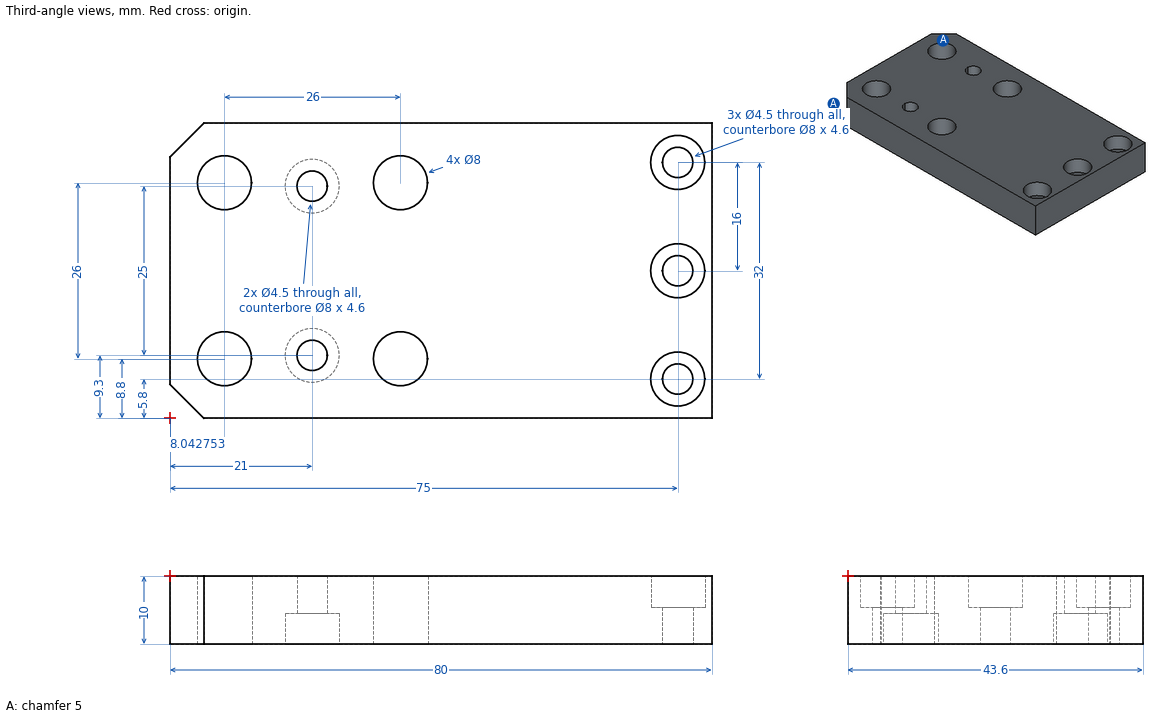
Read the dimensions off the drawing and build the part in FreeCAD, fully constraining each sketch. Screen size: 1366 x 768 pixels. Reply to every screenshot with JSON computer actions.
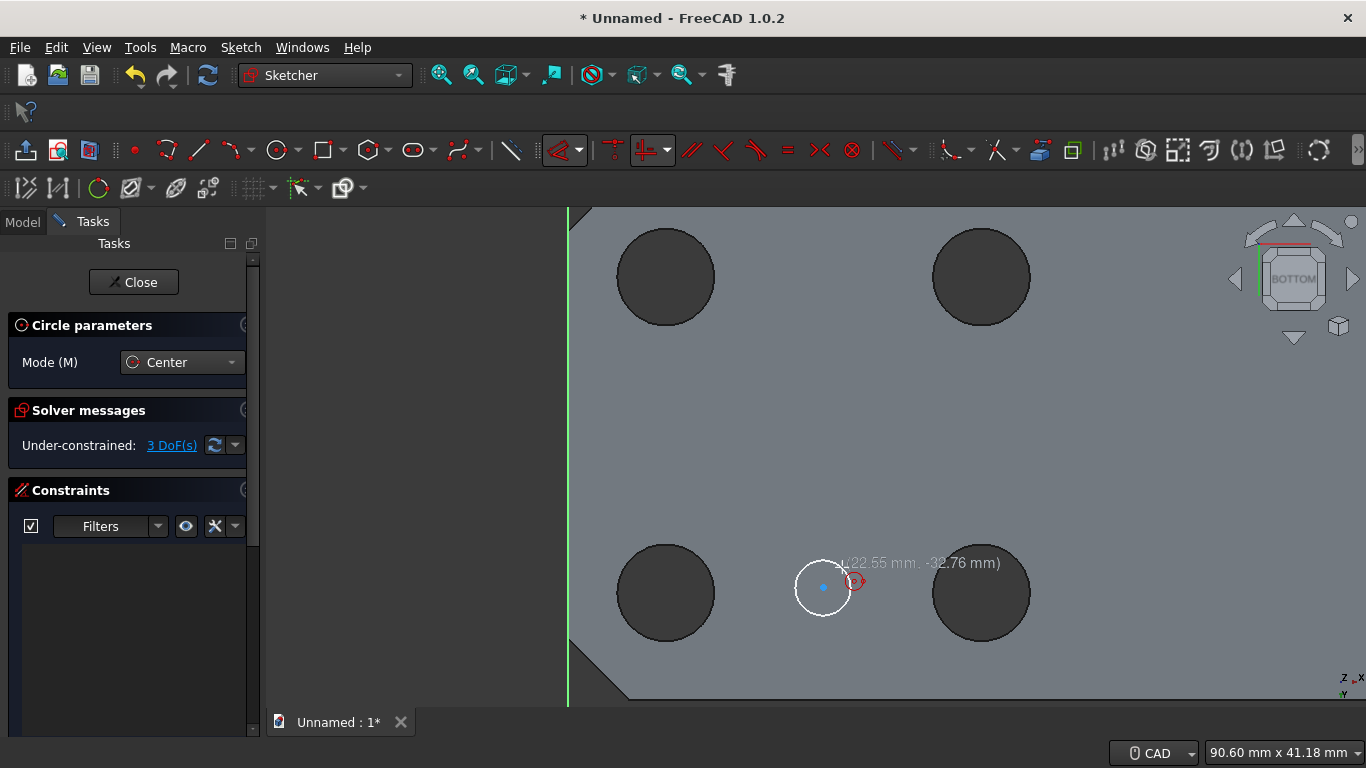
{"action": "left_click", "coordinate": [823, 283]}
{"action": "left_click", "coordinate": [842, 264]}
{"action": "key", "text": "Escape"}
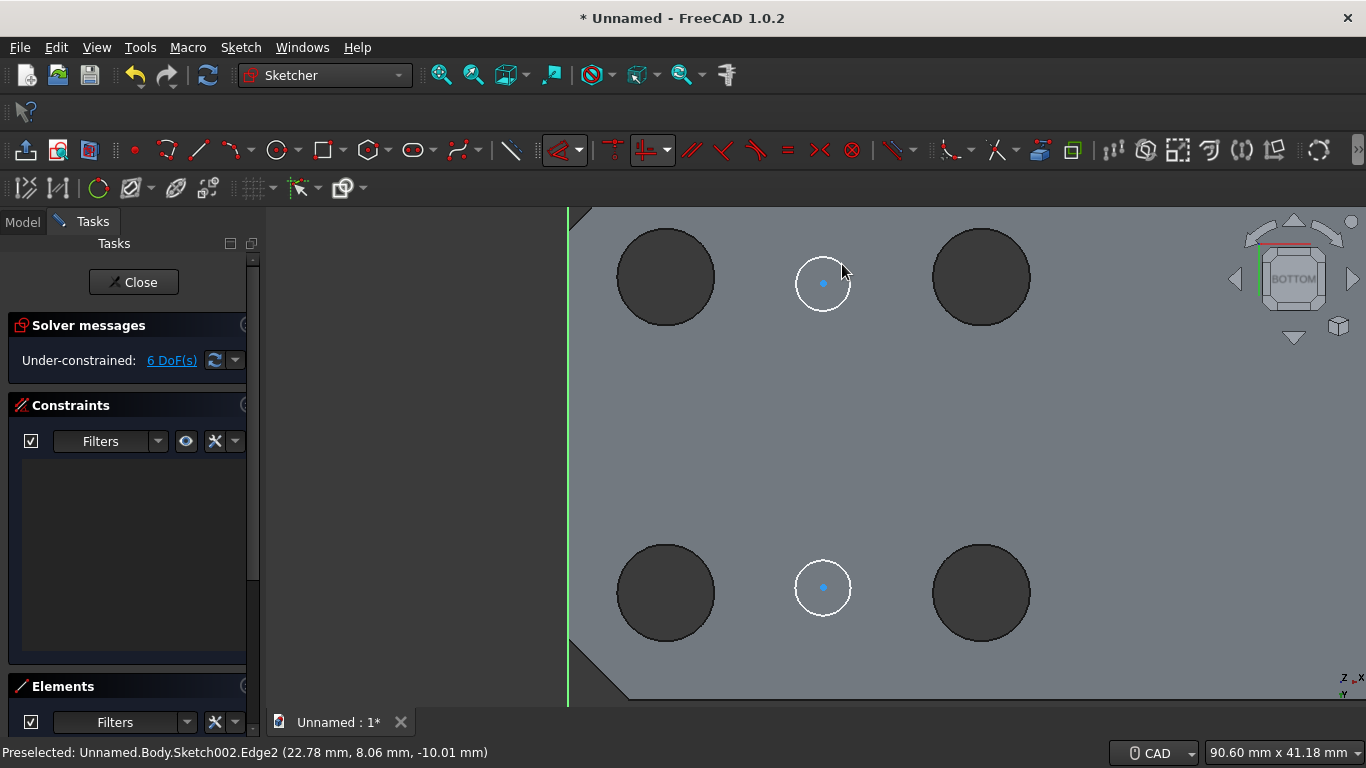
{"action": "left_click", "coordinate": [842, 568]}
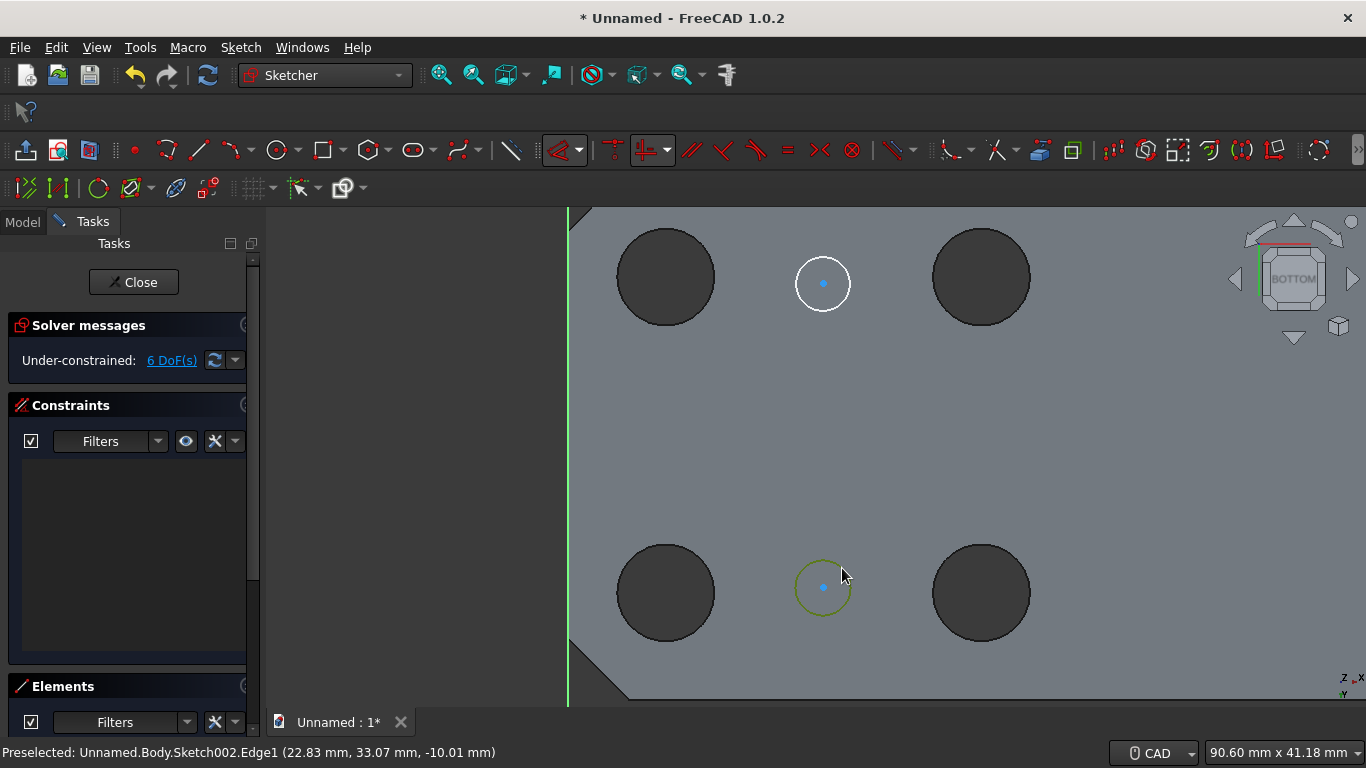
{"action": "left_click", "coordinate": [842, 265]}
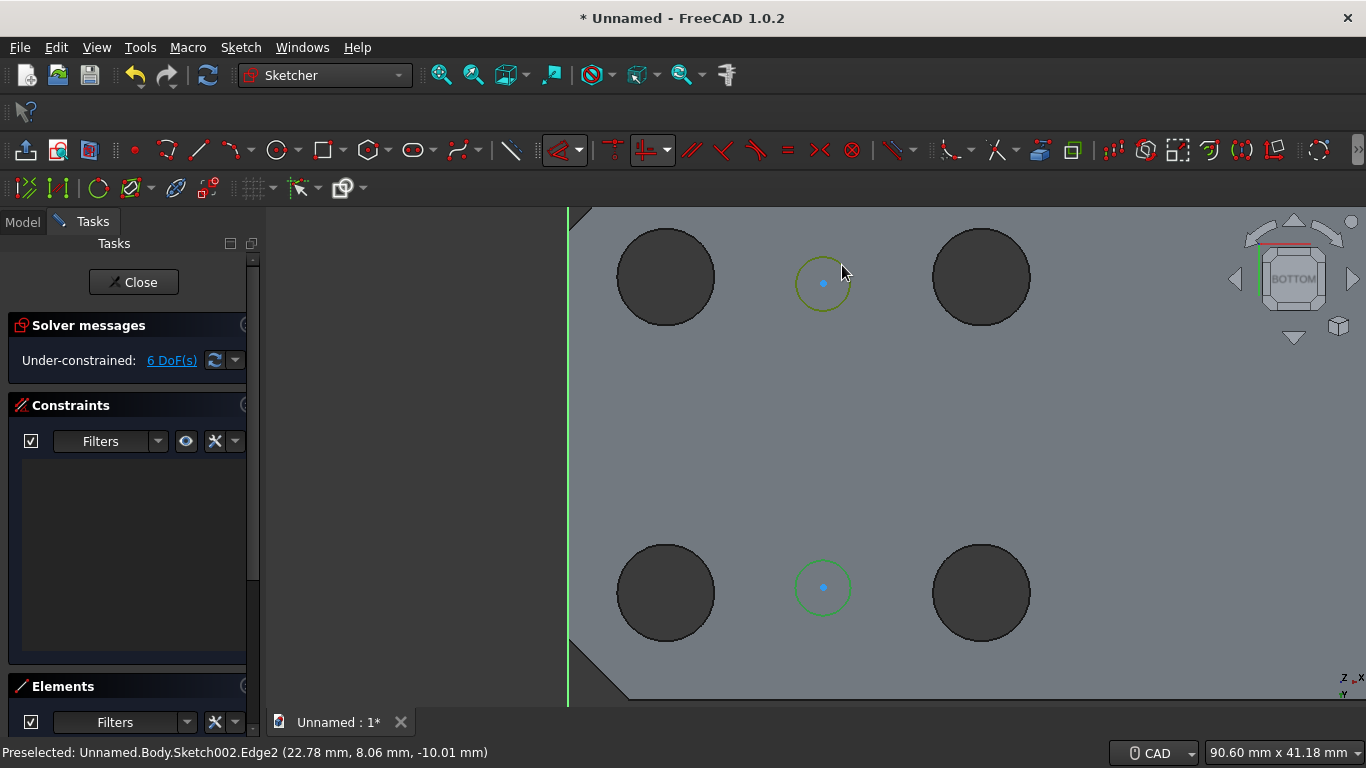
{"action": "left_click", "coordinate": [788, 150]}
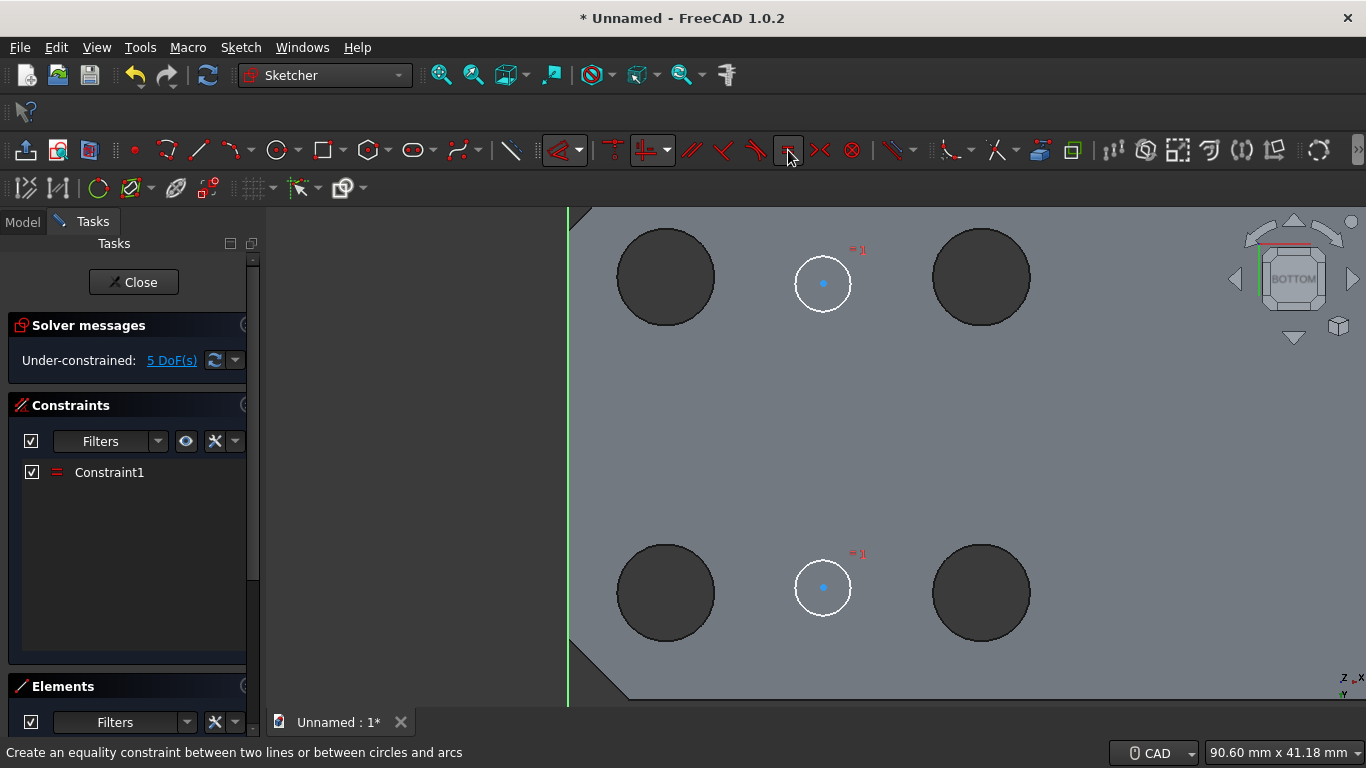
{"action": "left_click", "coordinate": [842, 568]}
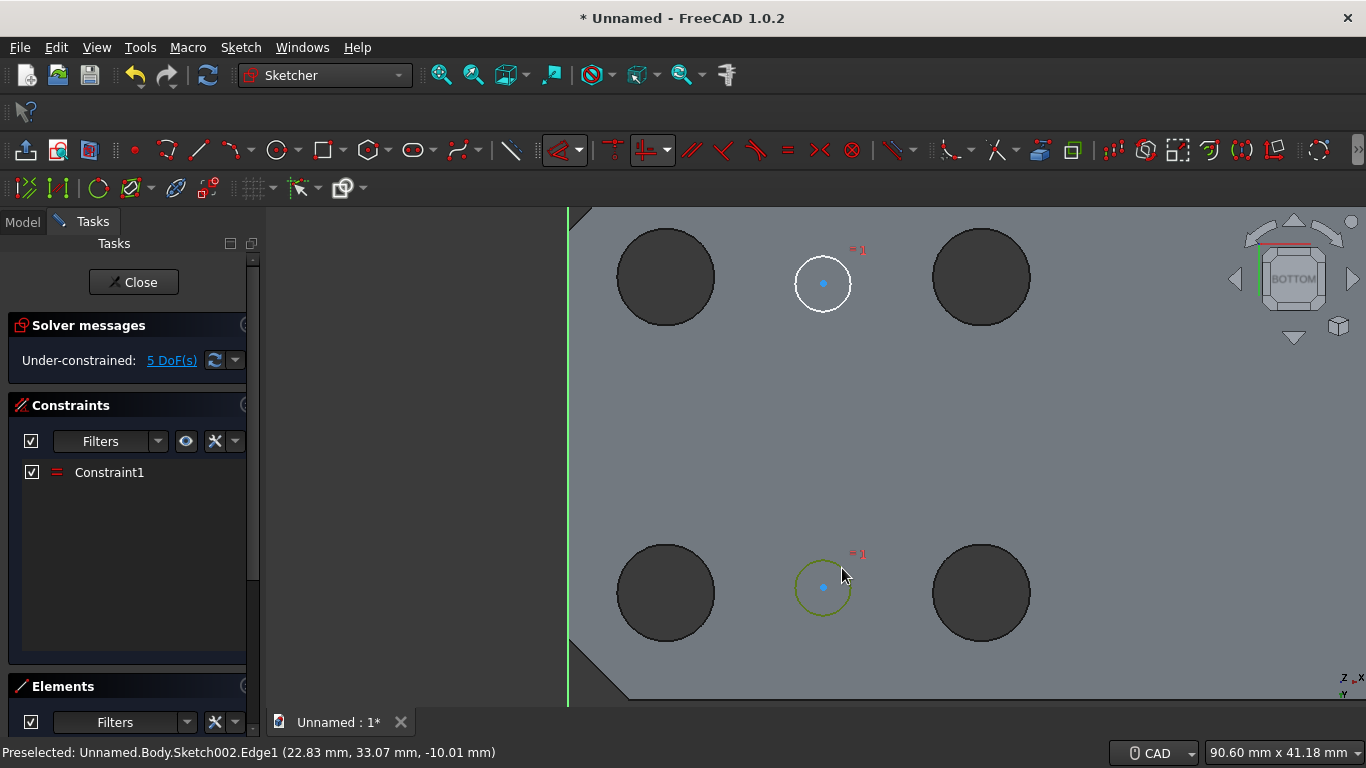
{"action": "left_click", "coordinate": [582, 150]}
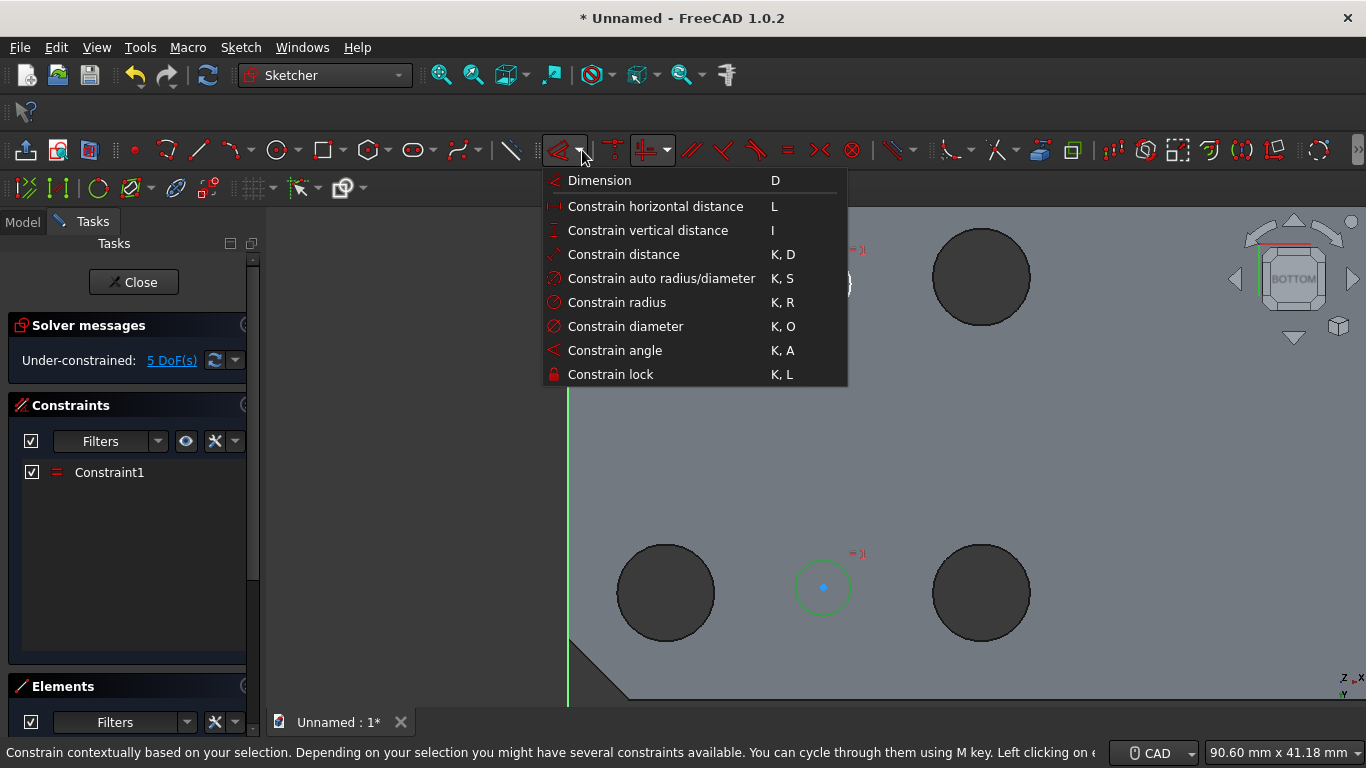
{"action": "left_click", "coordinate": [695, 326]}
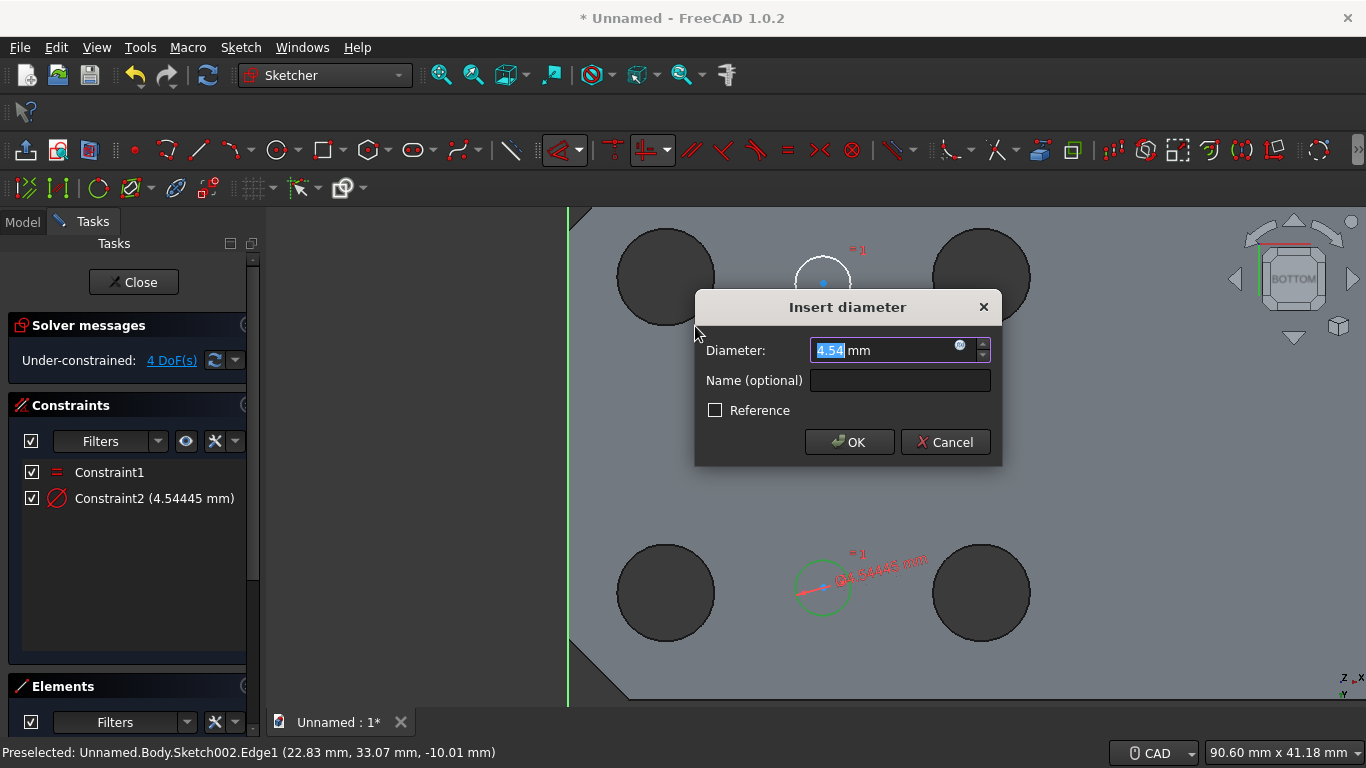
{"action": "type", "text": "4.5"}
{"action": "key", "text": "Return"}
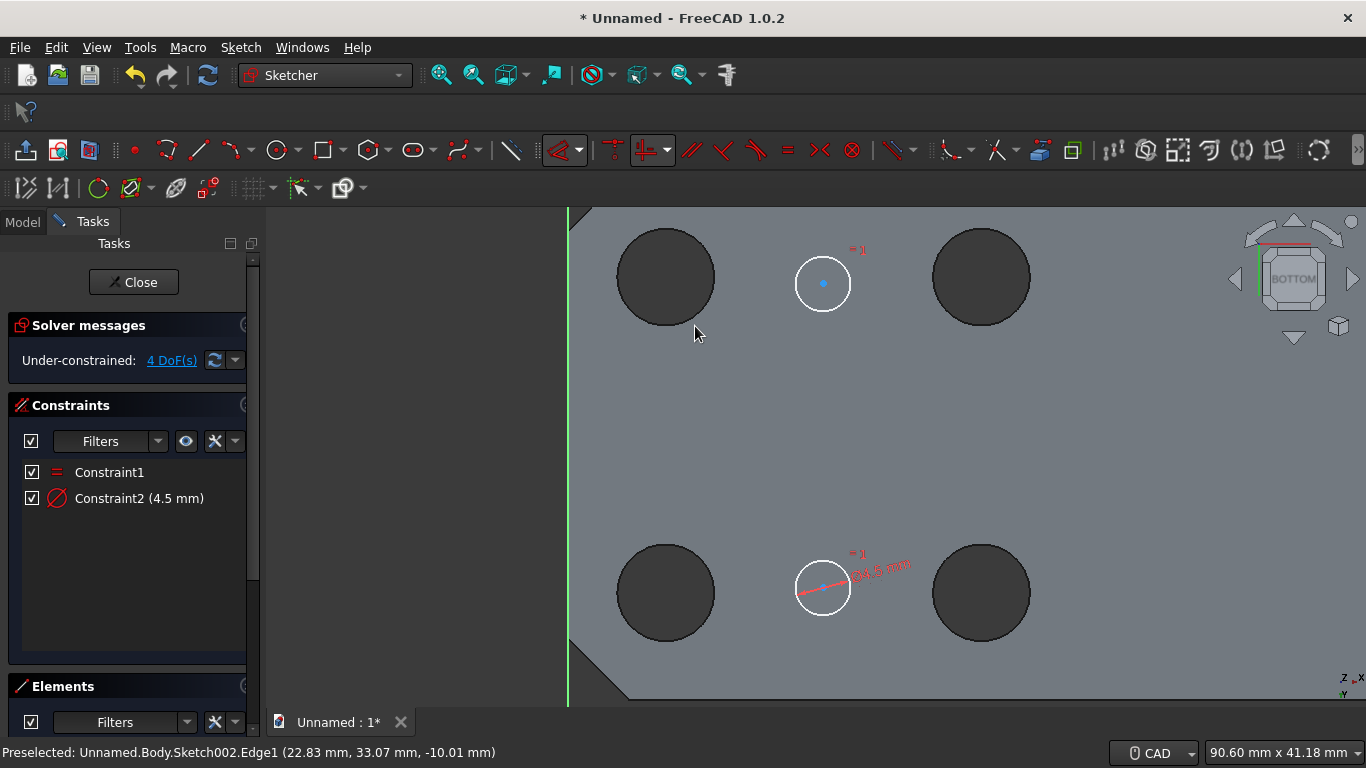
{"action": "left_click", "coordinate": [823, 588]}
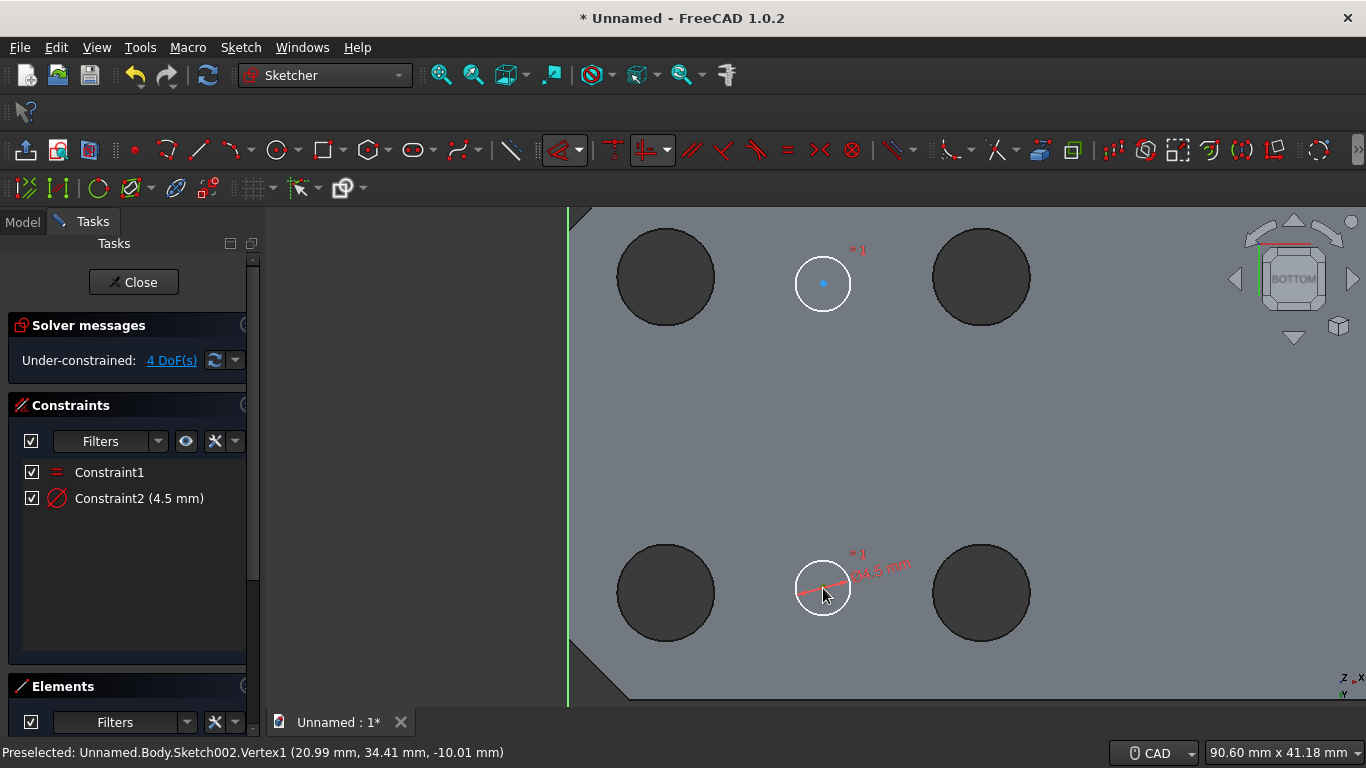
{"action": "left_click", "coordinate": [582, 150]}